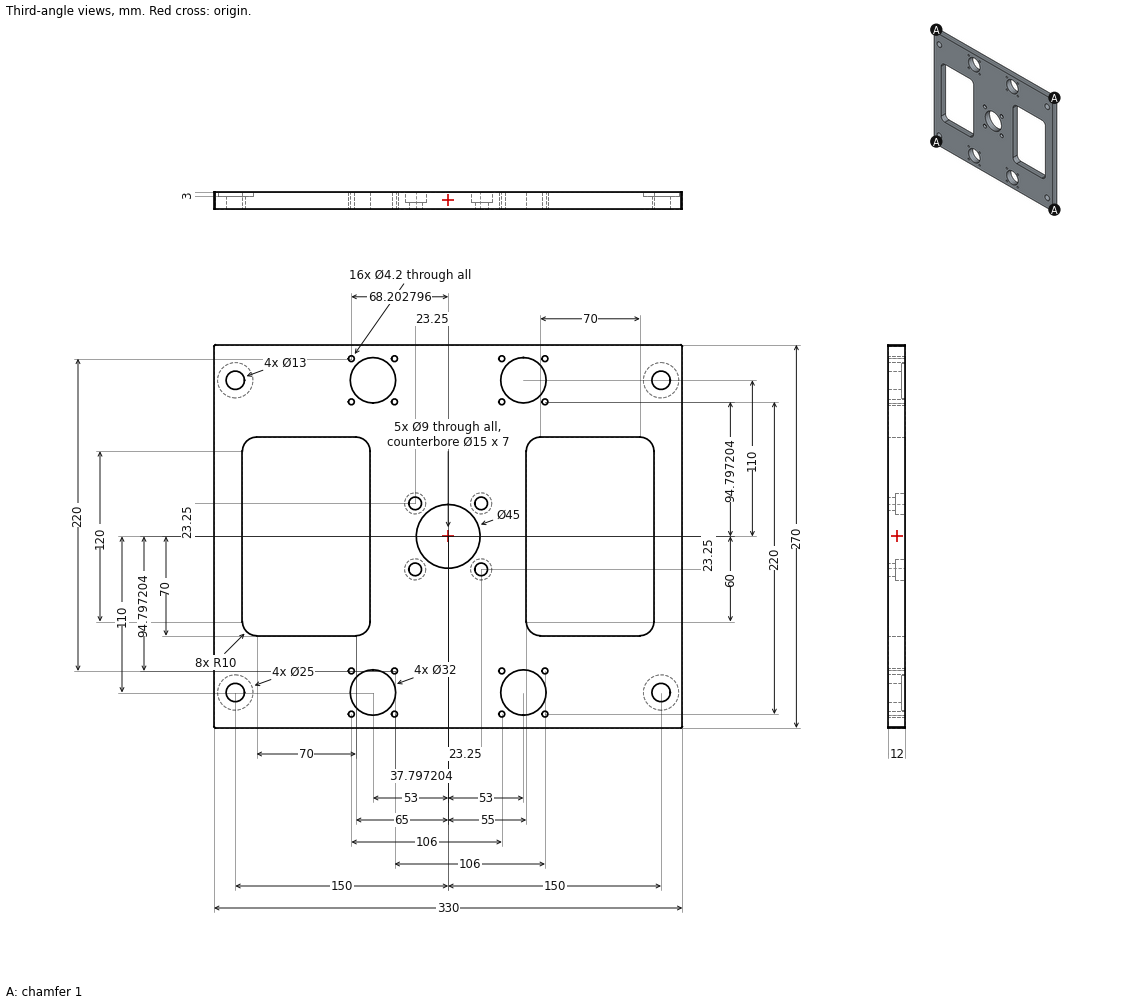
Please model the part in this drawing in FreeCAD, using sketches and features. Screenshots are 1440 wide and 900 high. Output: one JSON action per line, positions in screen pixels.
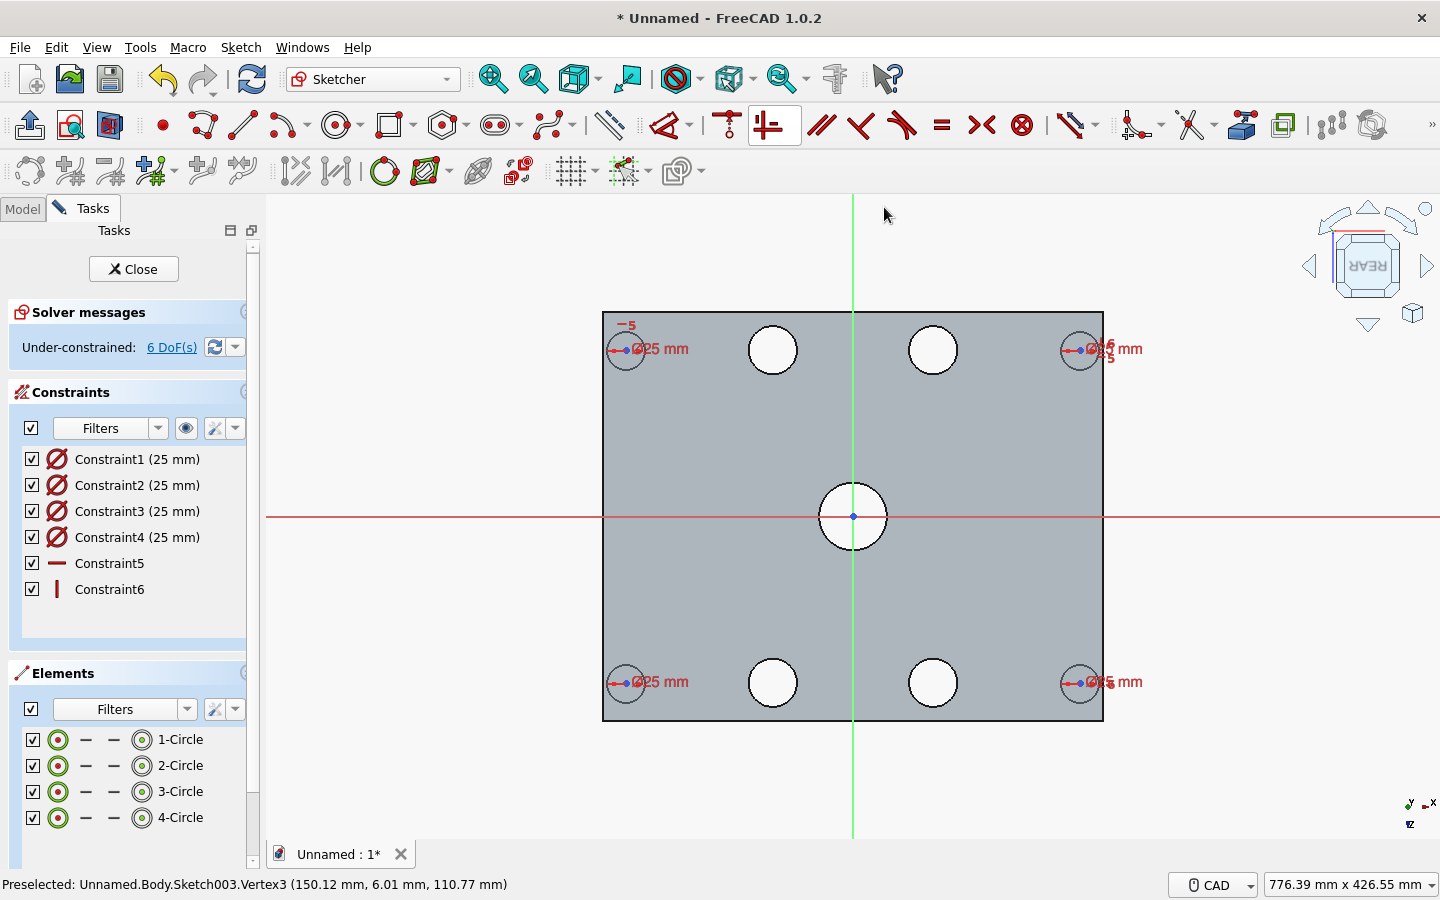
{"action": "left_click", "coordinate": [626, 351]}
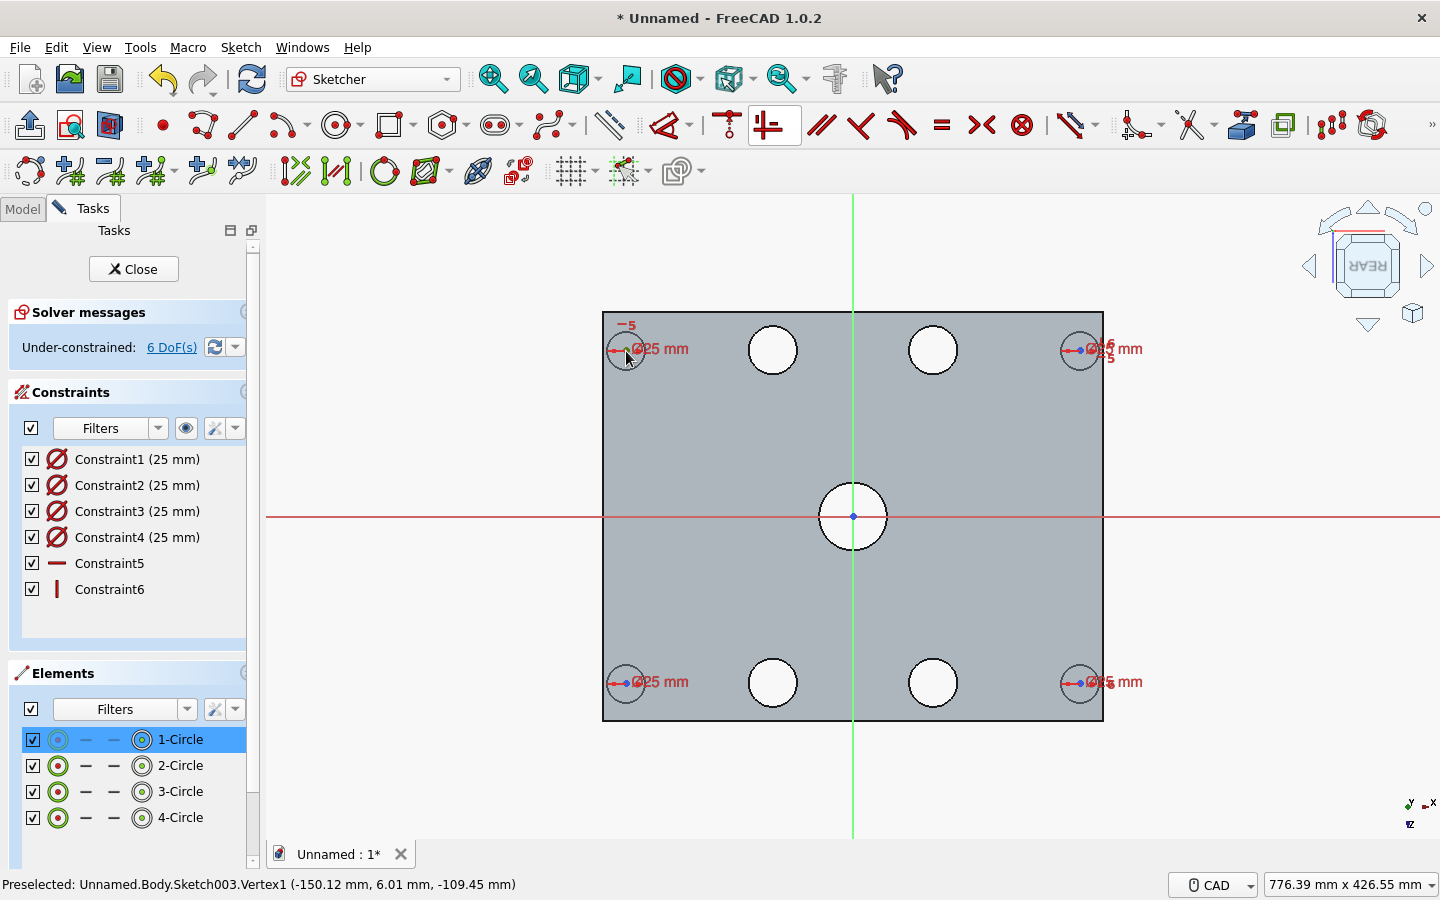
{"action": "left_click", "coordinate": [626, 684]}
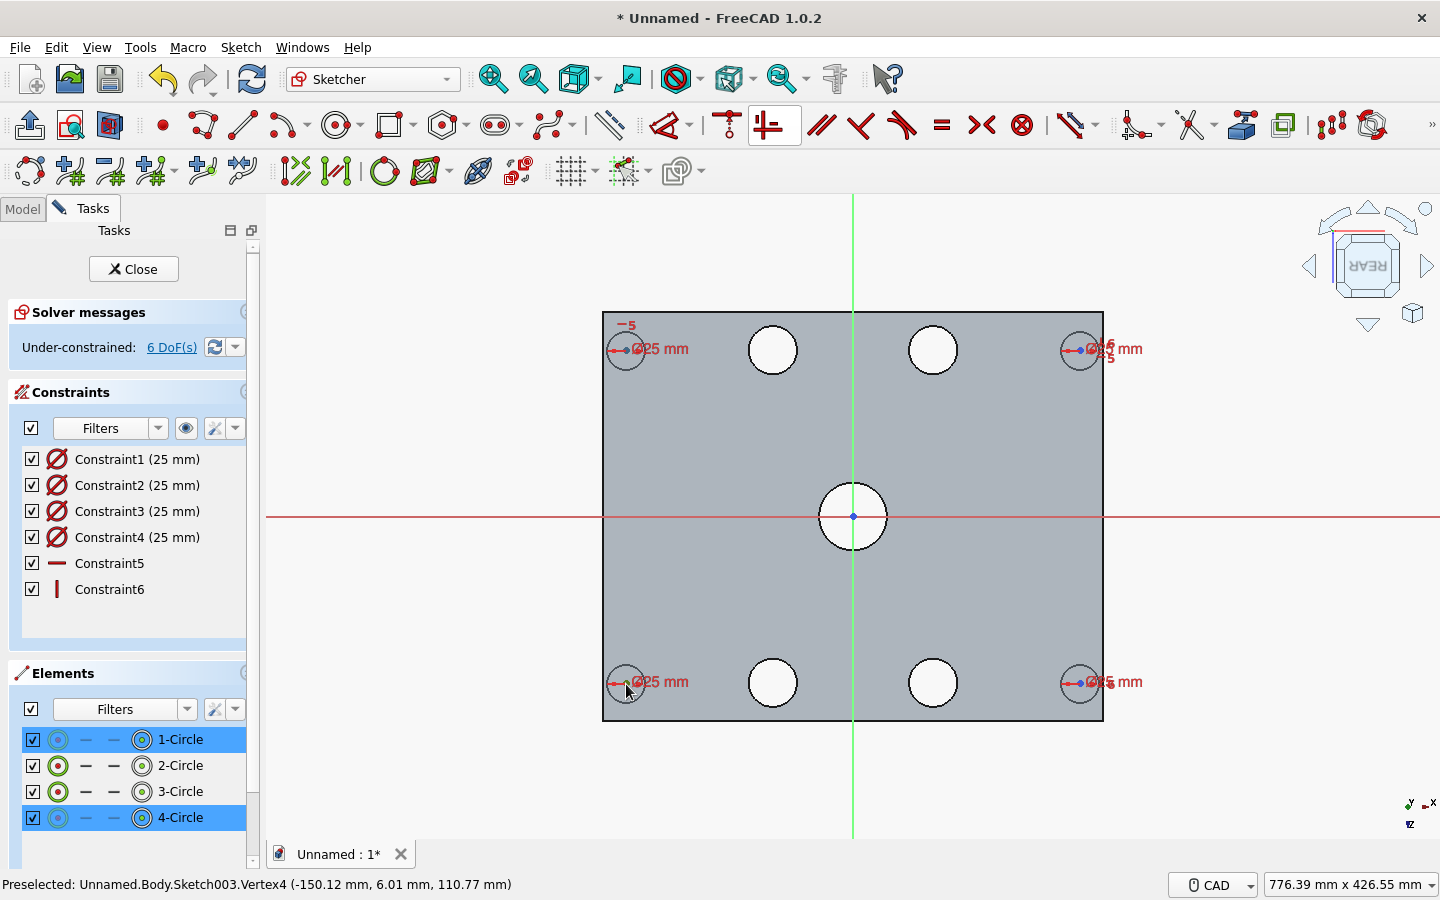
{"action": "left_click", "coordinate": [796, 126]}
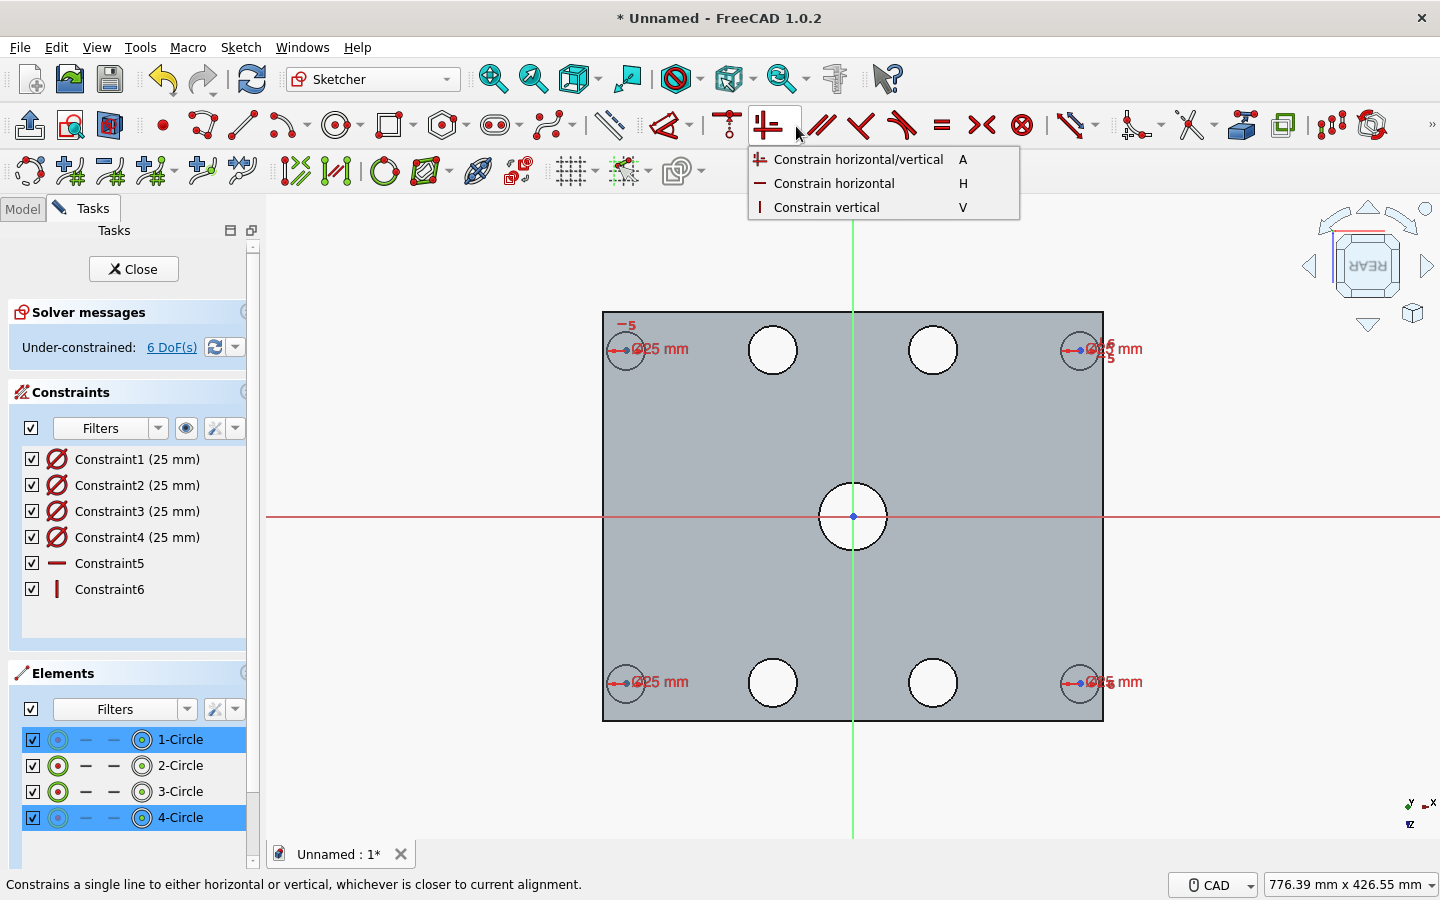
{"action": "left_click", "coordinate": [884, 207]}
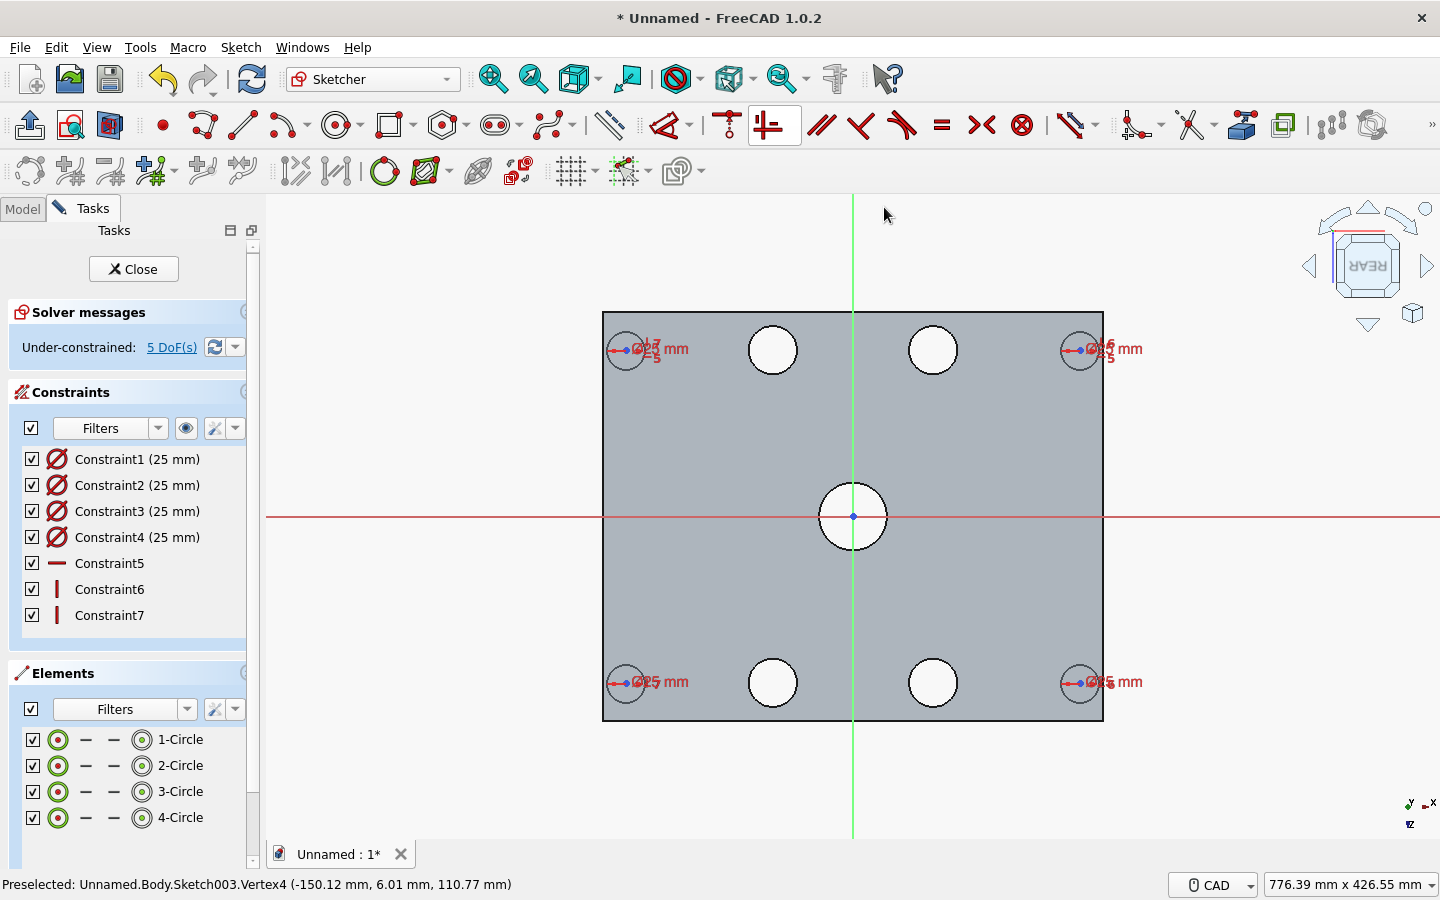
{"action": "left_click", "coordinate": [1080, 684]}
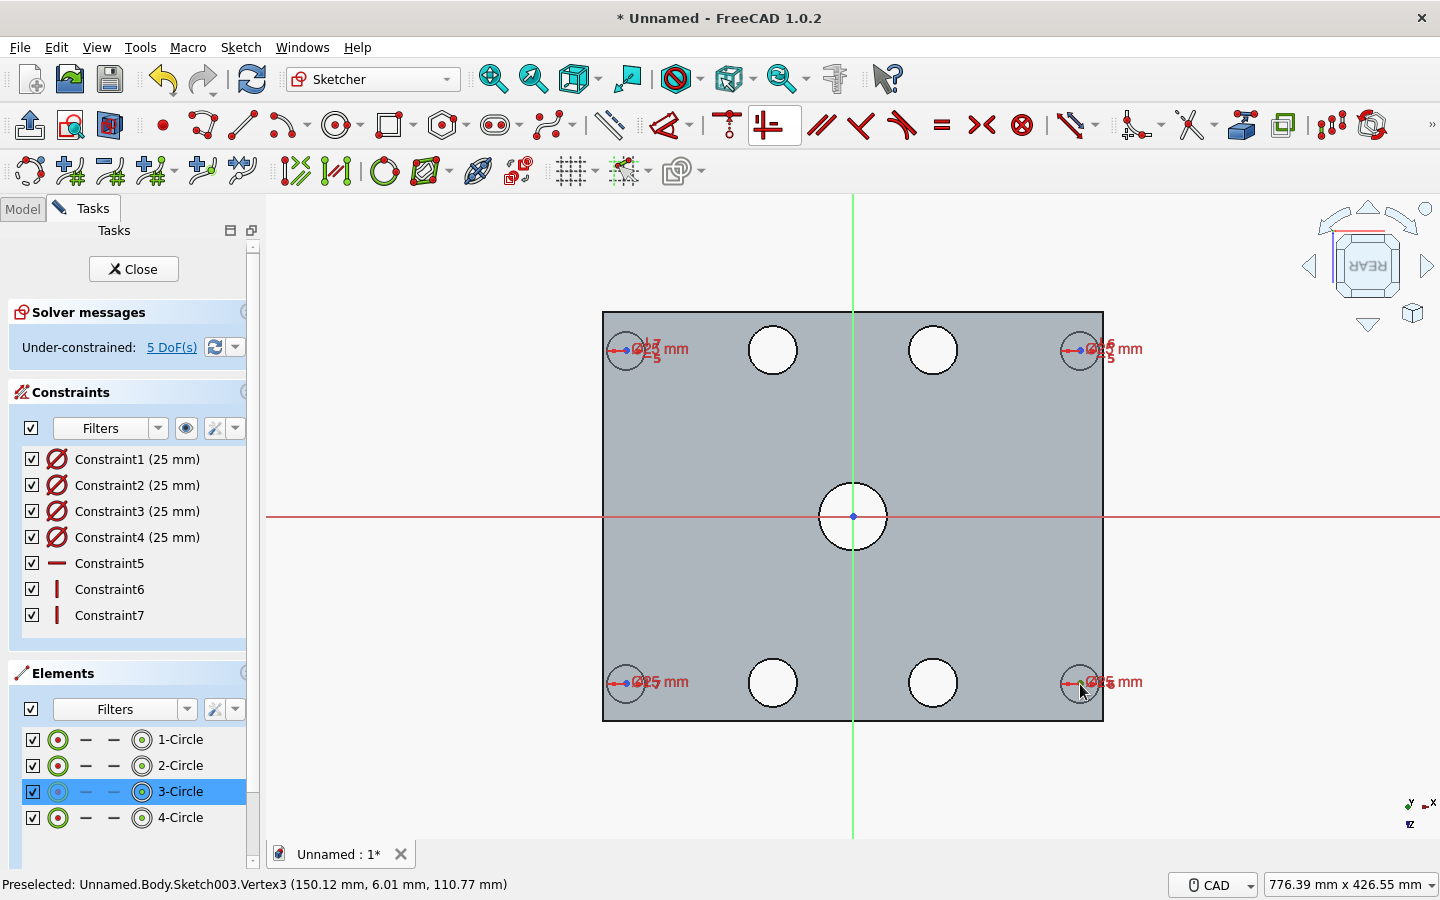
{"action": "left_click", "coordinate": [626, 684]}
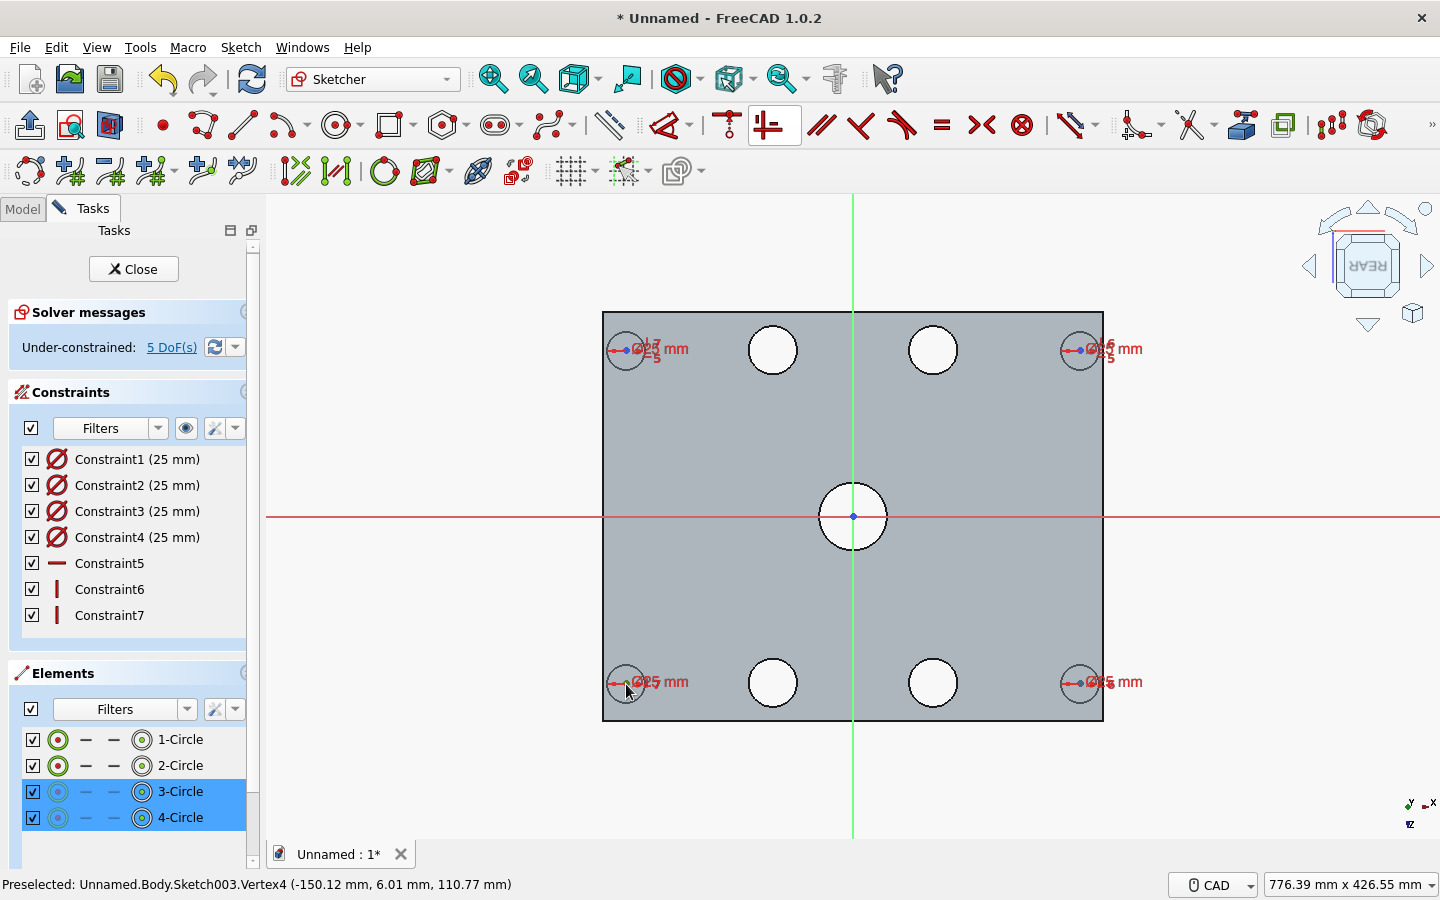
{"action": "left_click", "coordinate": [796, 126]}